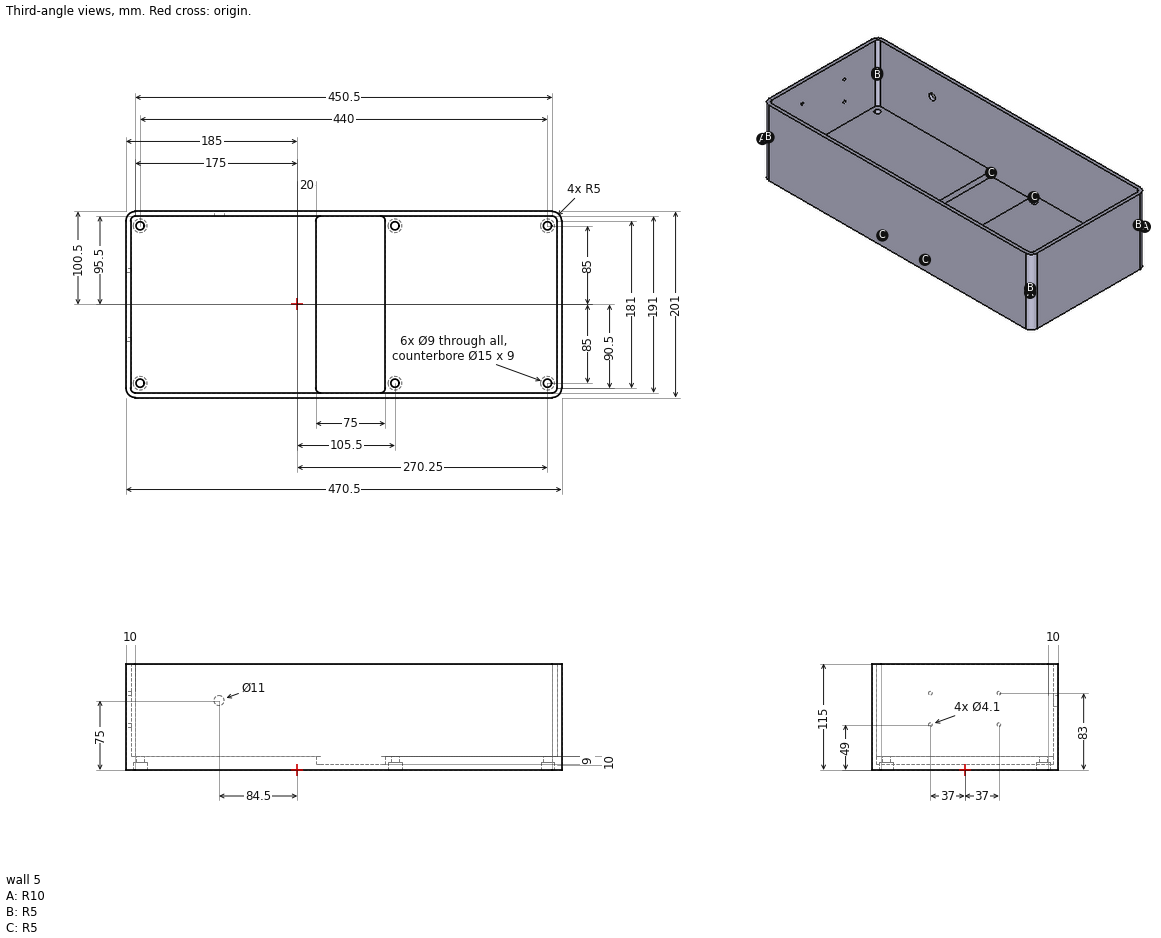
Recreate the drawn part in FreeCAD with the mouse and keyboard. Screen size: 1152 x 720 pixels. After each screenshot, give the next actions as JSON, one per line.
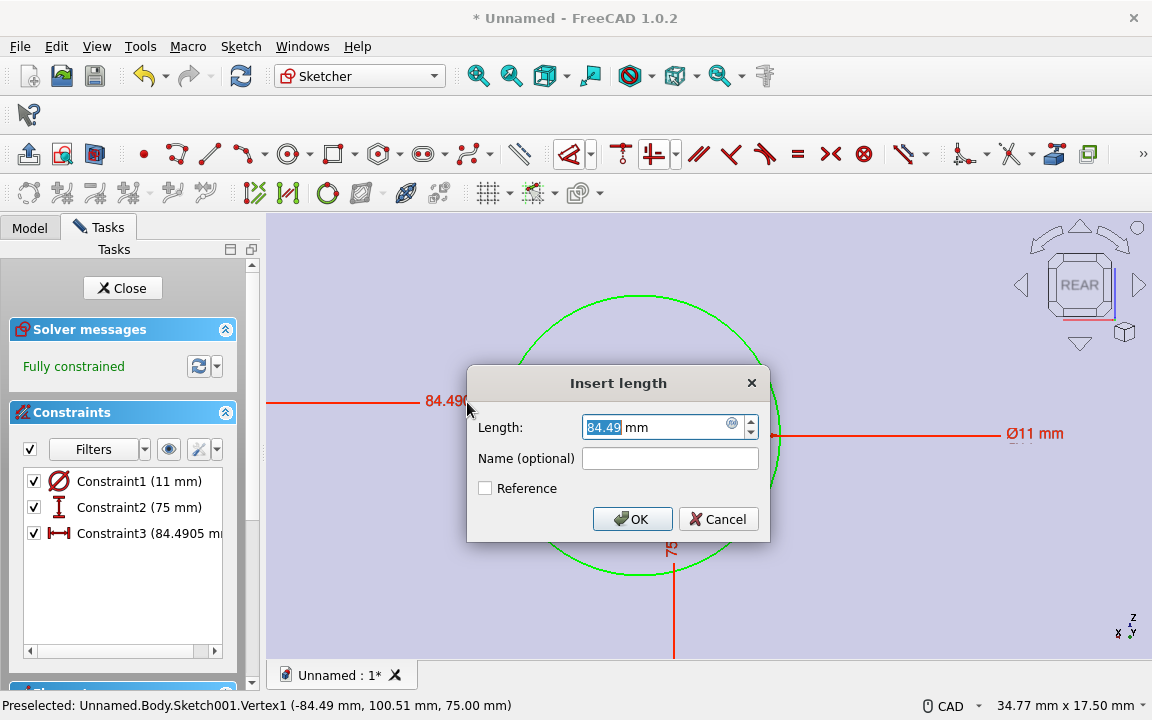
{"action": "type", "text": "84.5"}
{"action": "key", "text": "Return"}
{"action": "key", "text": "Escape"}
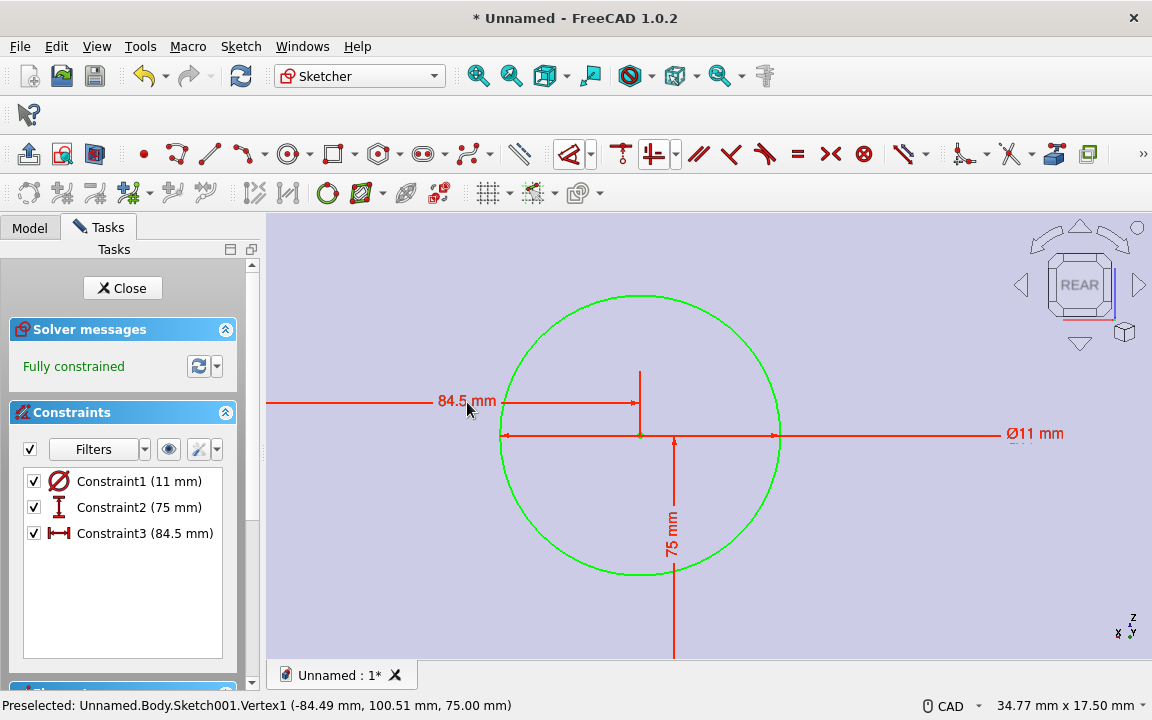
{"action": "left_click", "coordinate": [123, 288]}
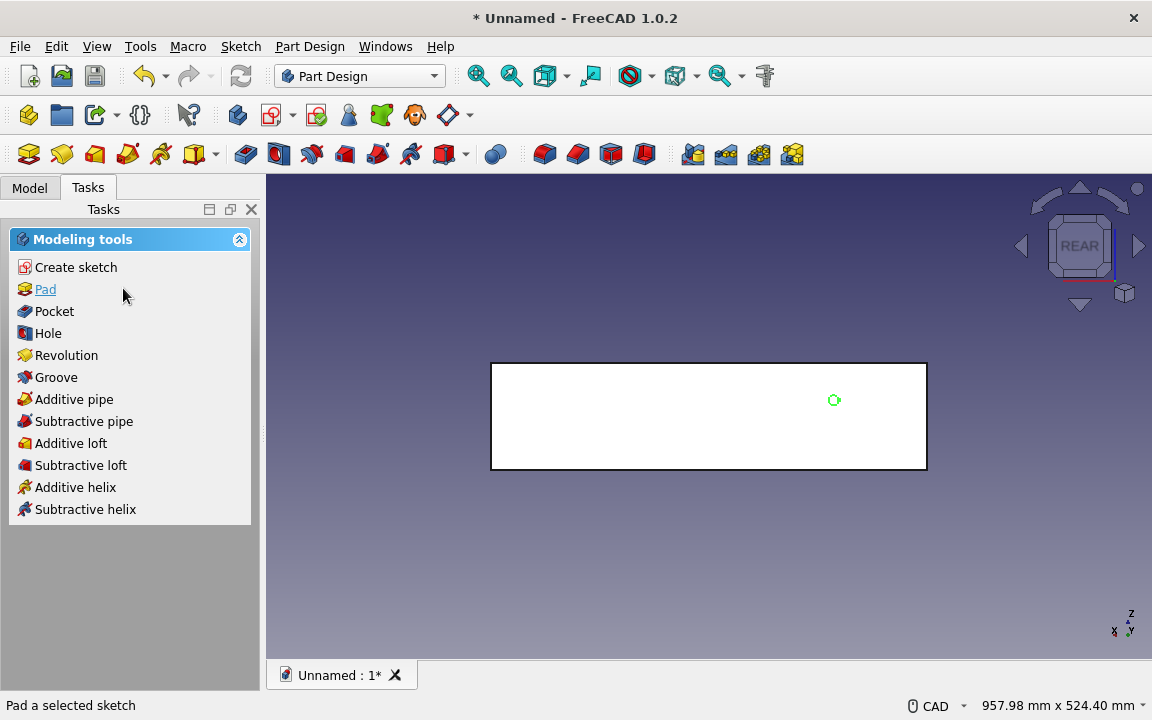
{"action": "left_click", "coordinate": [246, 154]}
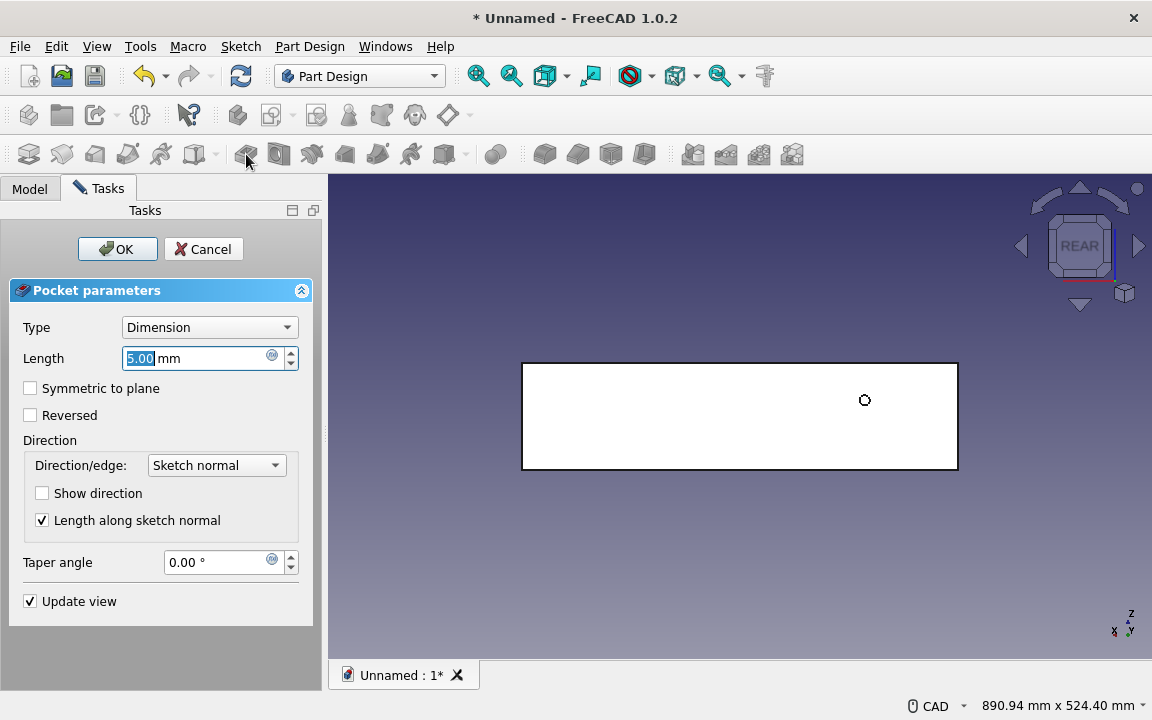
{"action": "type", "text": "10"}
{"action": "key", "text": "Tab"}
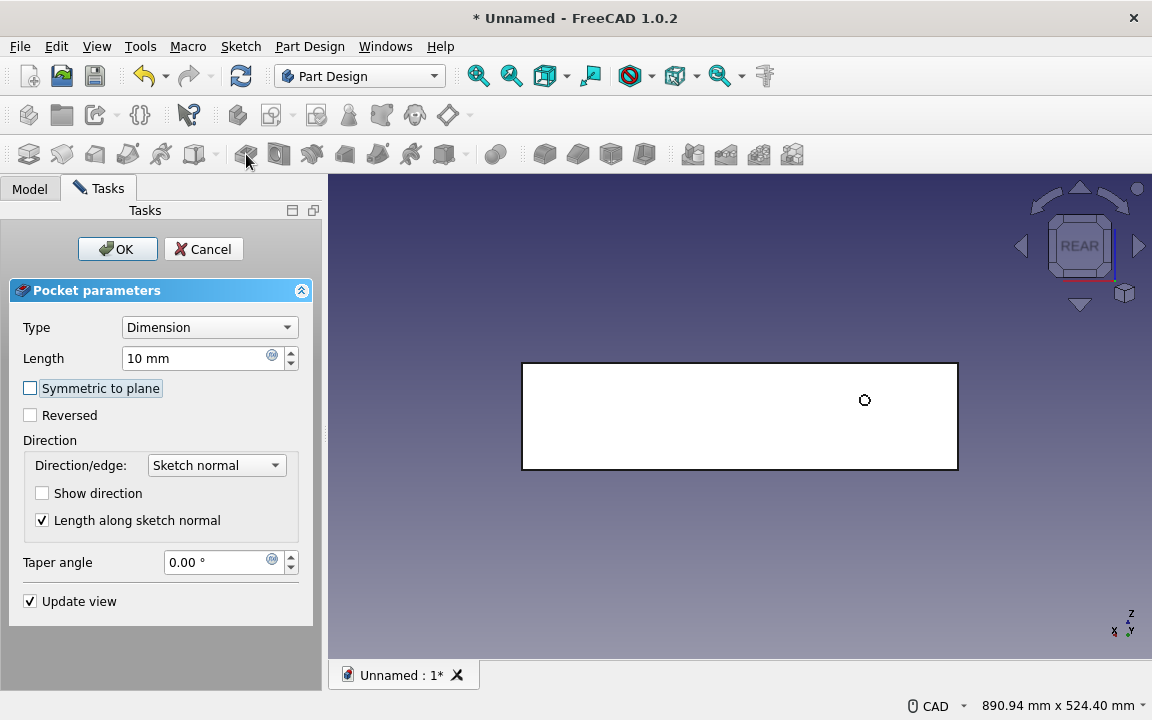
{"action": "left_click", "coordinate": [118, 249]}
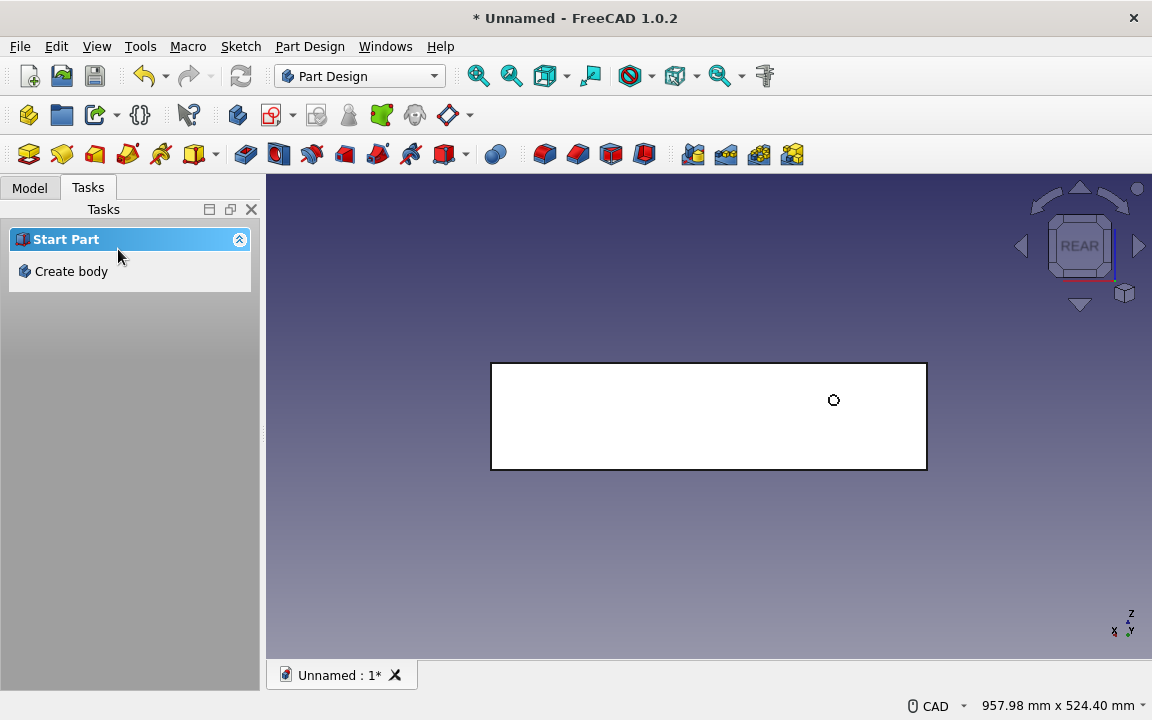
{"action": "key", "text": "6"}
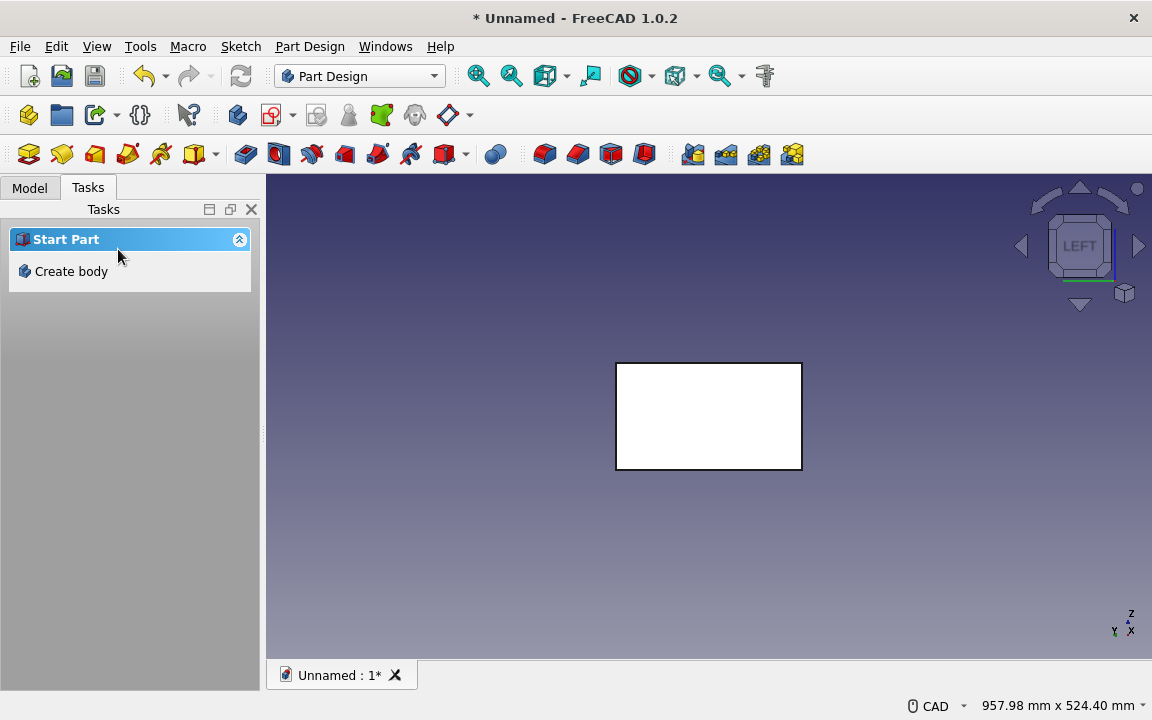
{"action": "key", "text": "v f"}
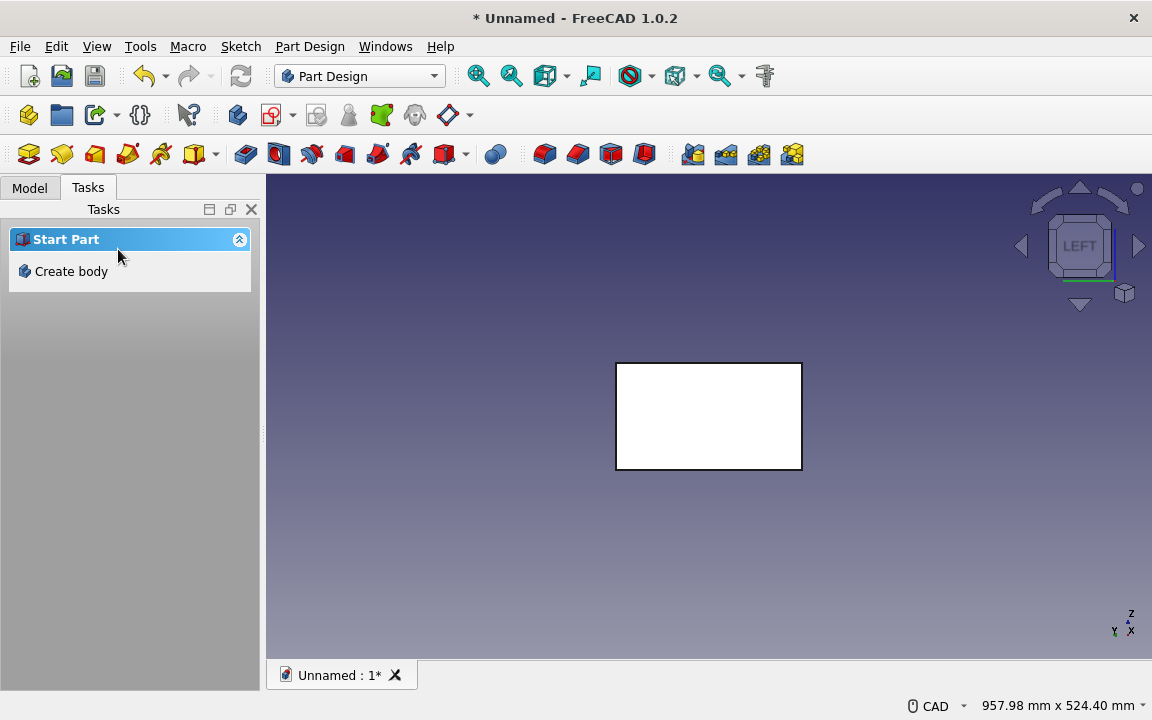
{"action": "left_click", "coordinate": [682, 415]}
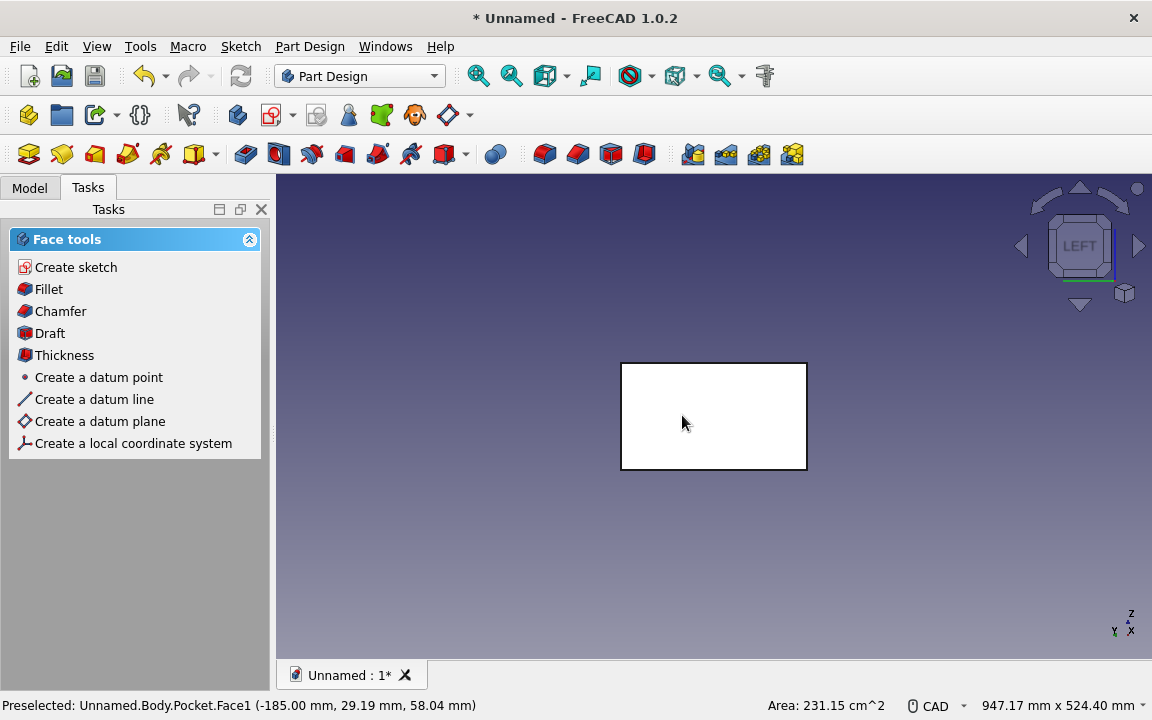
{"action": "left_click", "coordinate": [270, 116]}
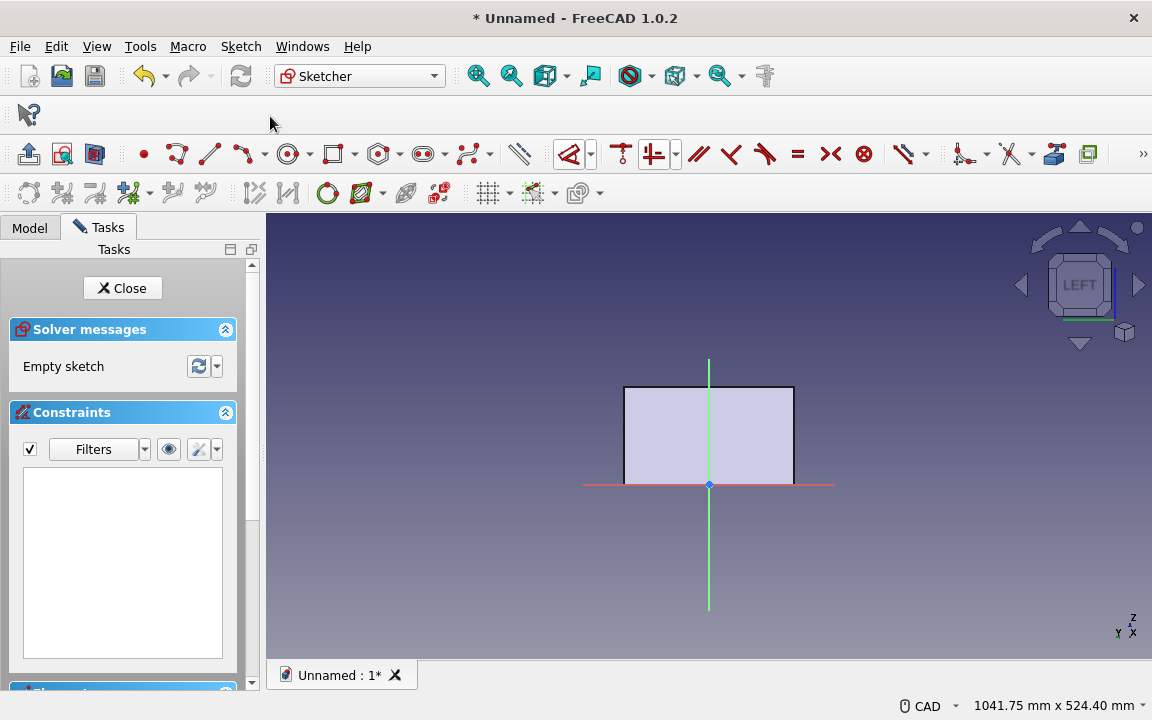
{"action": "scroll", "coordinate": [731, 453], "scroll_direction": "up", "scroll_amount": 7}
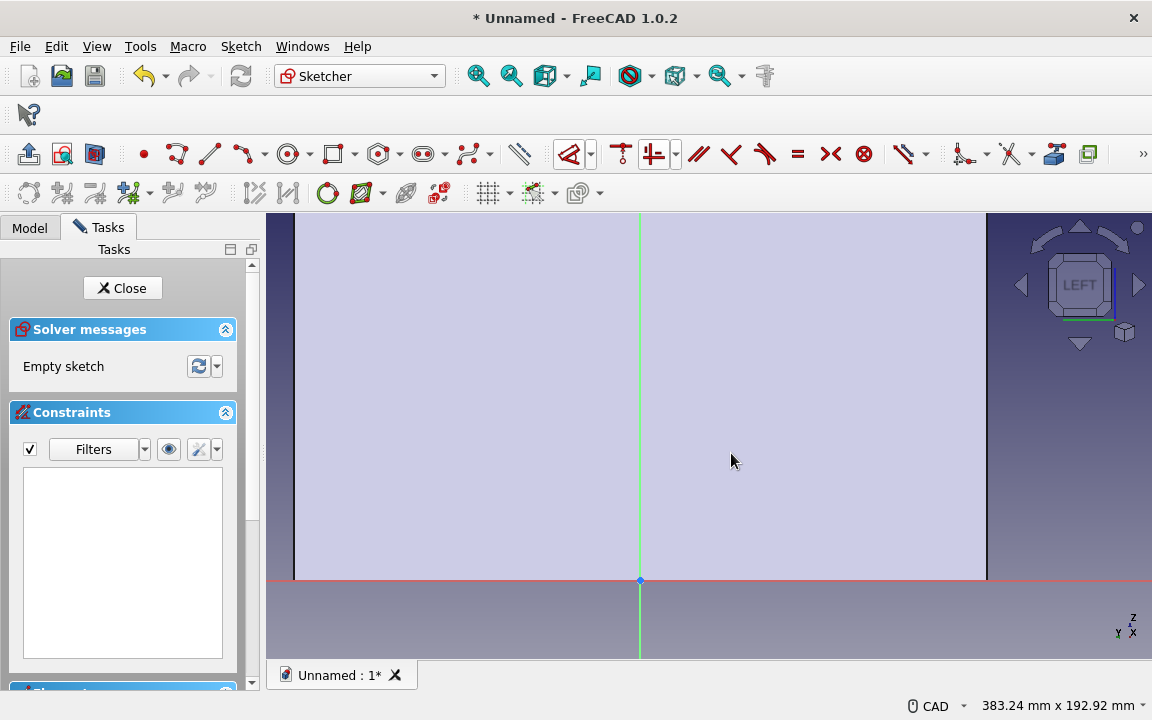
{"action": "left_click", "coordinate": [288, 154]}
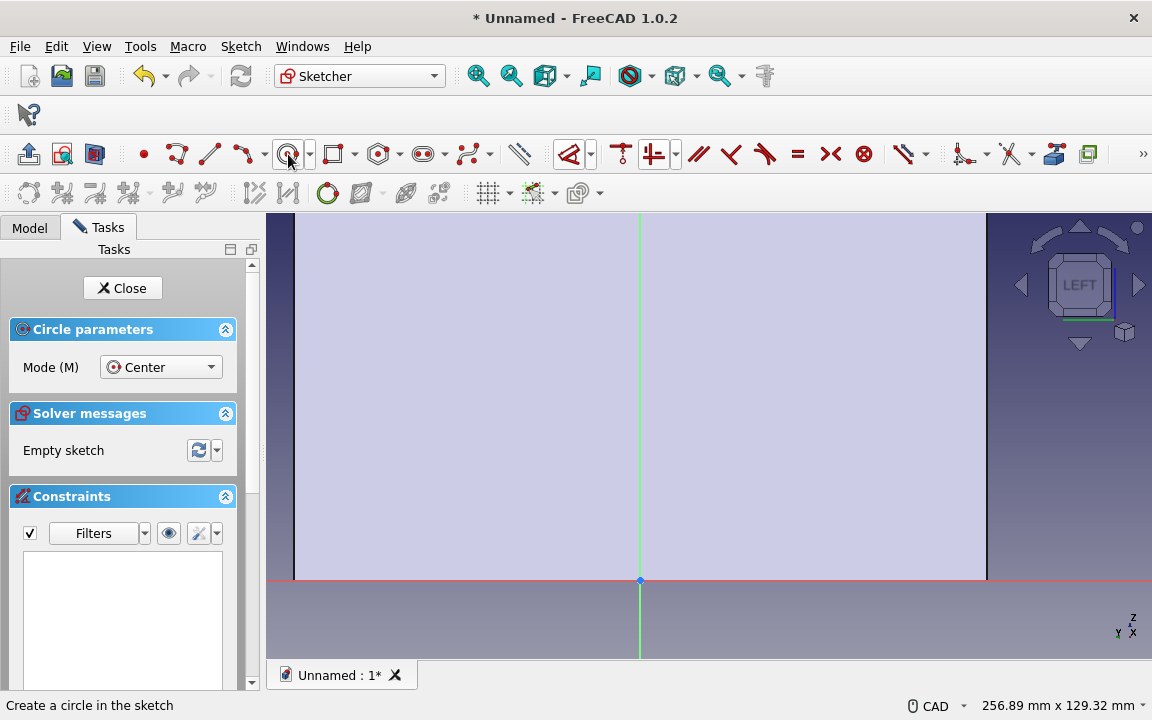
{"action": "scroll", "coordinate": [768, 412], "scroll_direction": "up", "scroll_amount": 6}